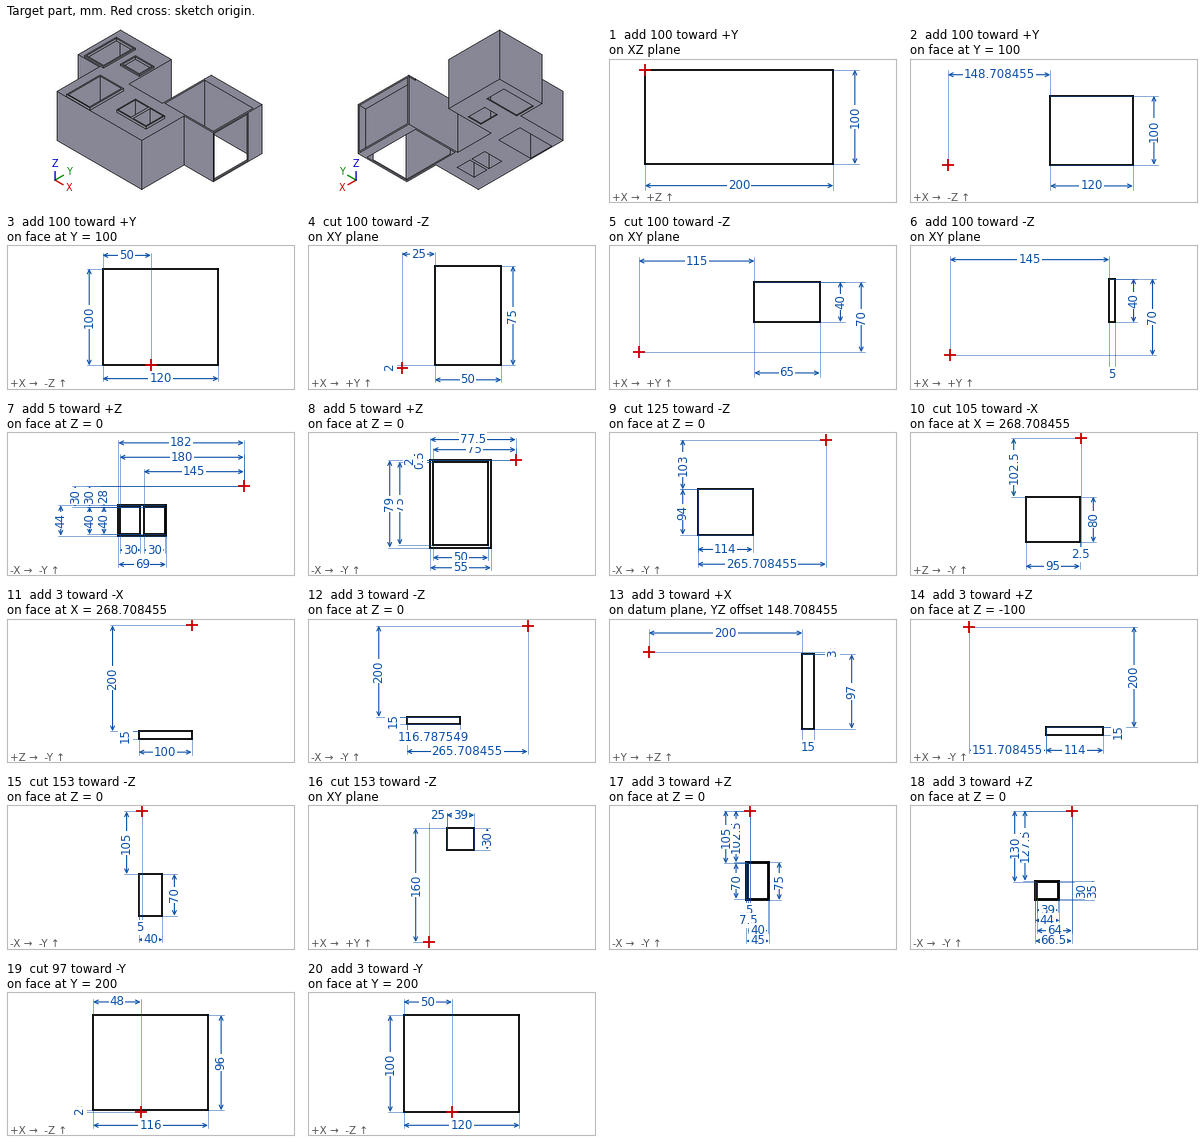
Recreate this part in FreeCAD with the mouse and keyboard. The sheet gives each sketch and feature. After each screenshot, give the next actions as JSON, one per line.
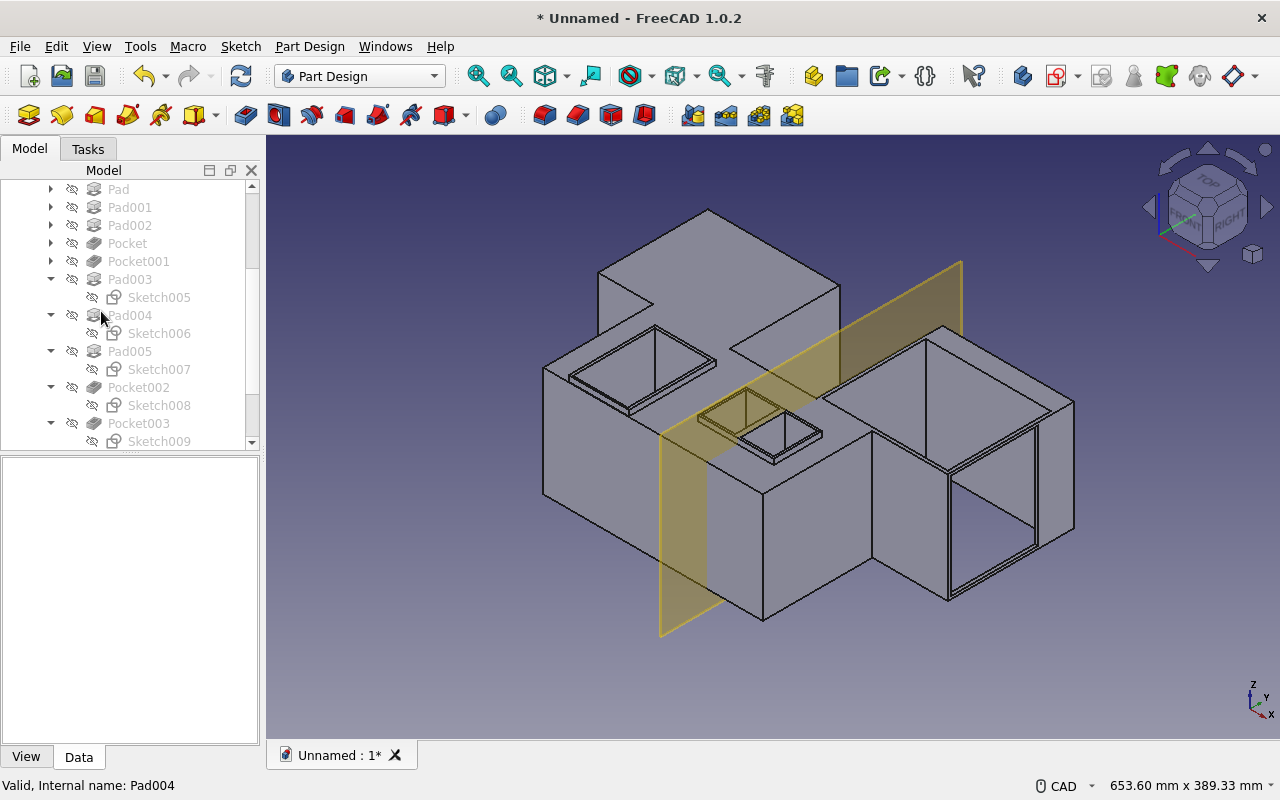
{"action": "scroll", "coordinate": [141, 311], "scroll_direction": "up", "scroll_amount": 15}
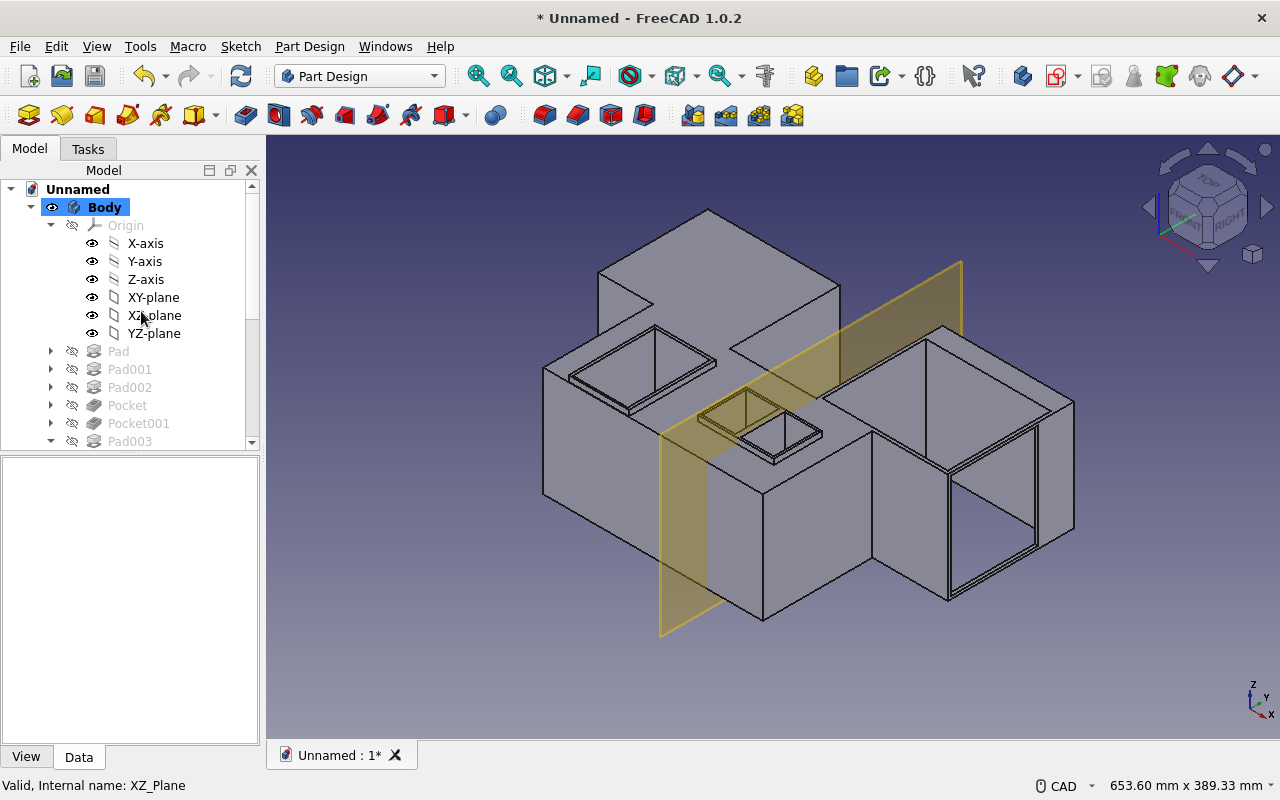
{"action": "scroll", "coordinate": [101, 311], "scroll_direction": "down", "scroll_amount": 6}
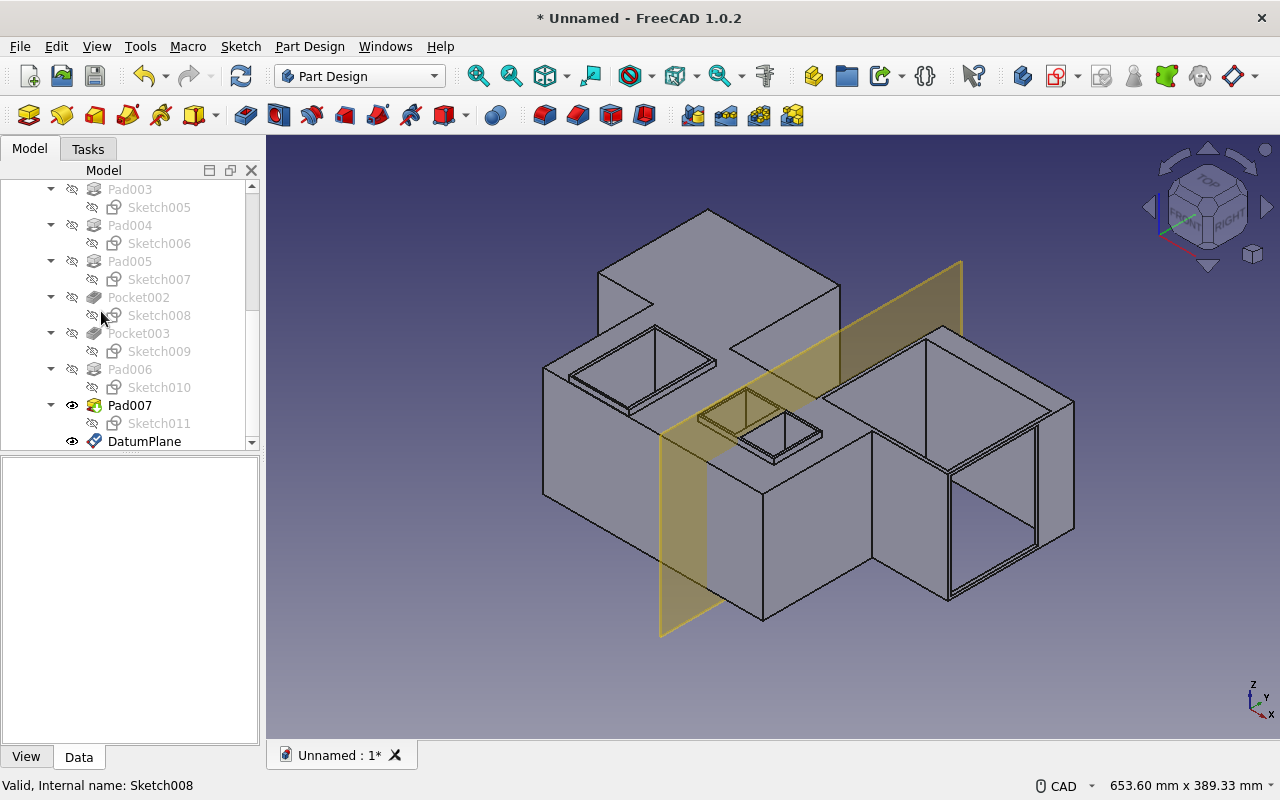
{"action": "left_click", "coordinate": [117, 441]}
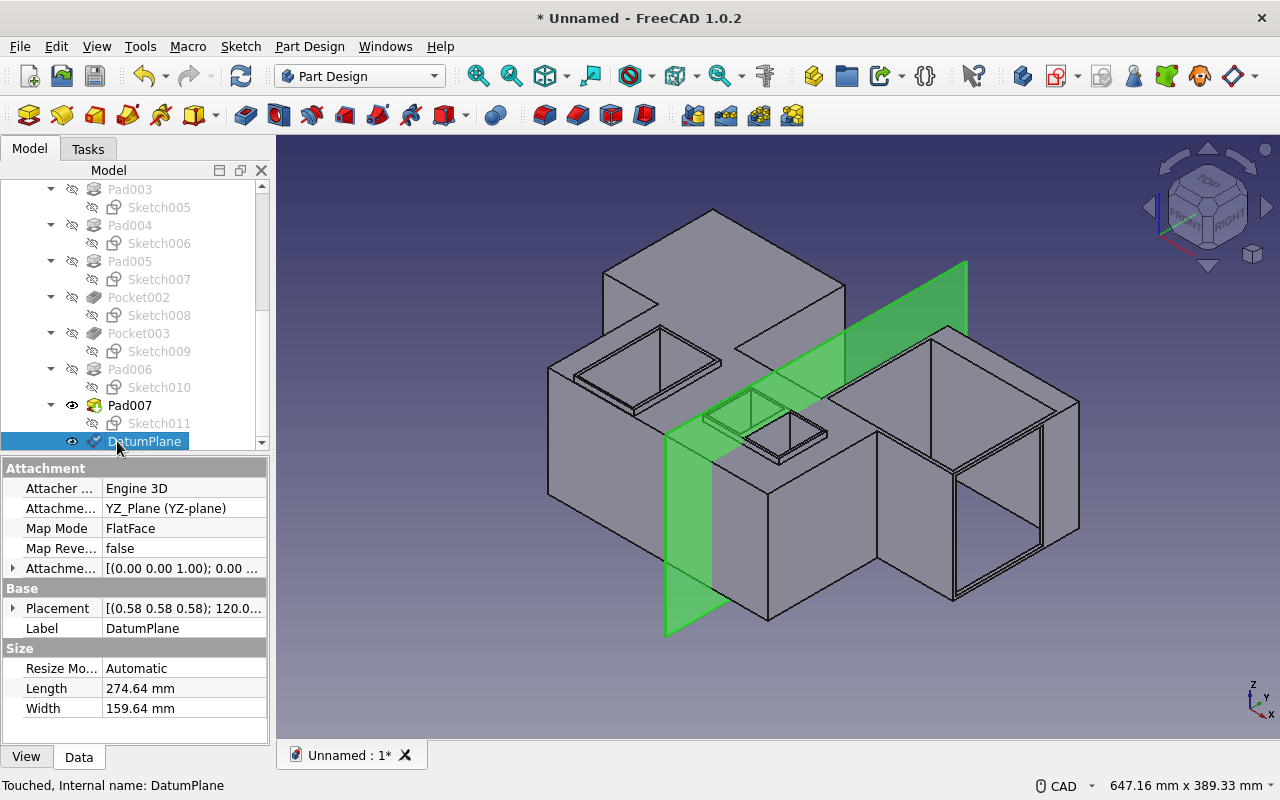
{"action": "left_click", "coordinate": [1056, 76]}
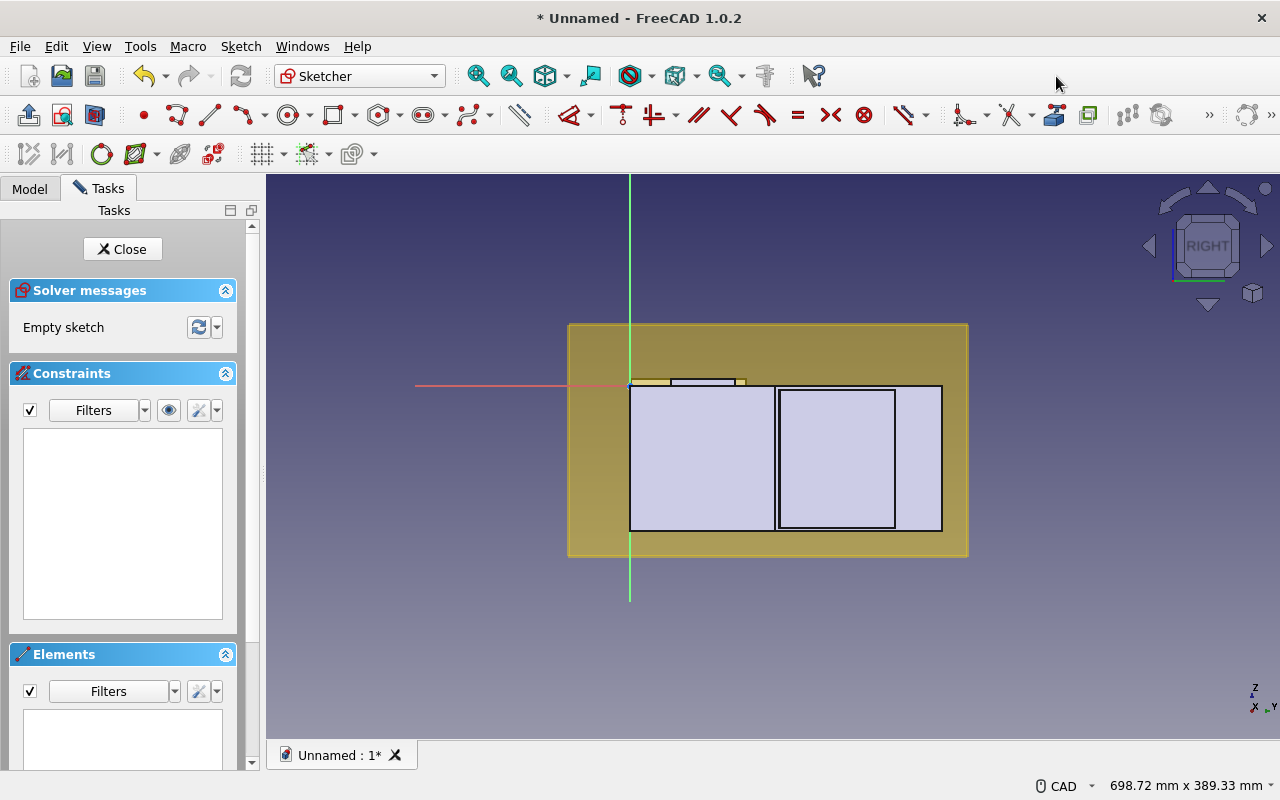
{"action": "left_click", "coordinate": [95, 116]}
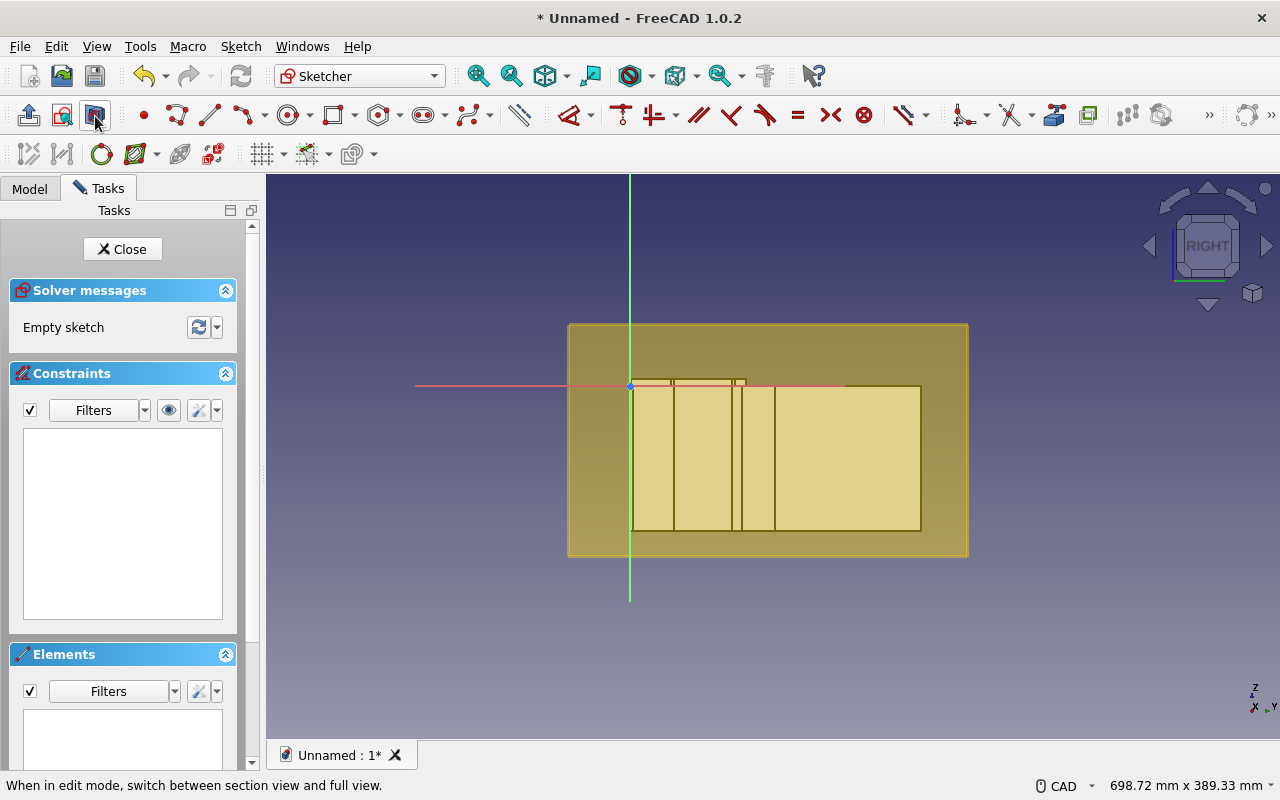
{"action": "scroll", "coordinate": [886, 462], "scroll_direction": "up", "scroll_amount": 3}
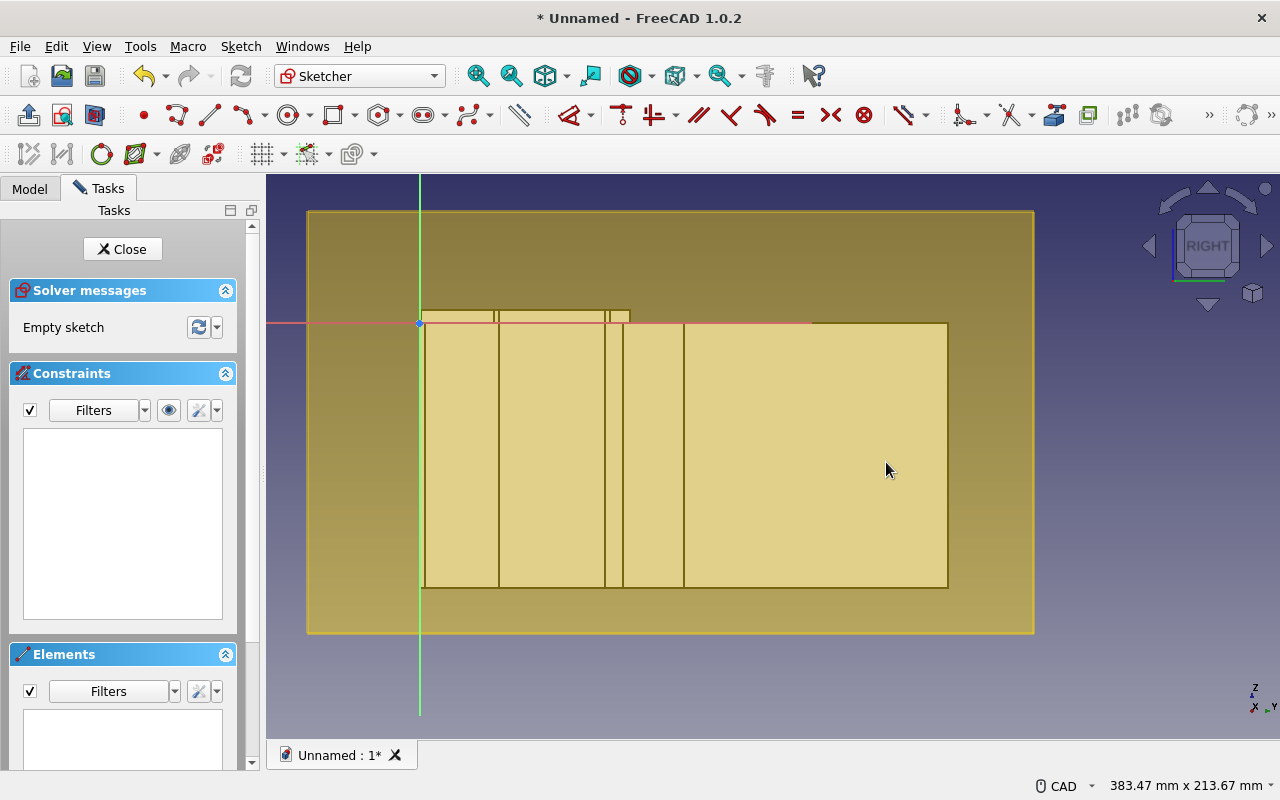
{"action": "left_click", "coordinate": [332, 116]}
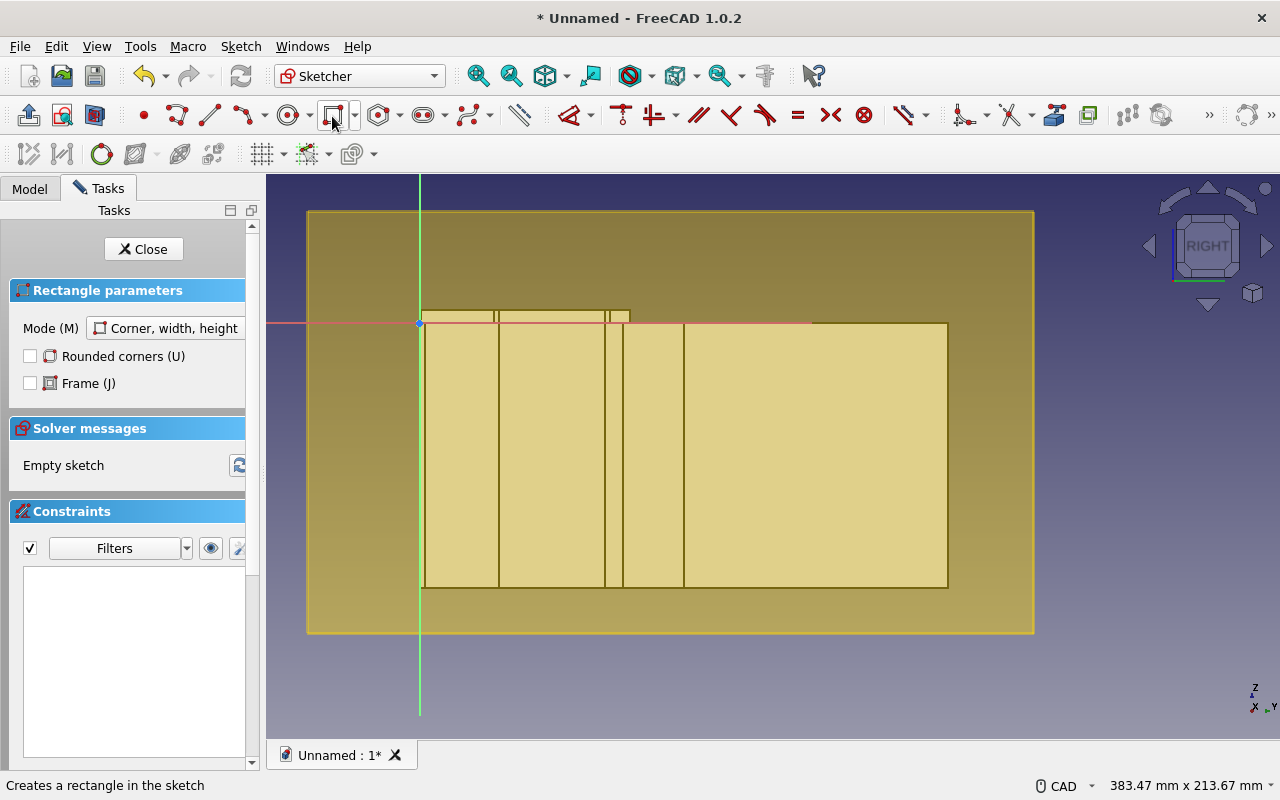
{"action": "scroll", "coordinate": [948, 331], "scroll_direction": "up", "scroll_amount": 4}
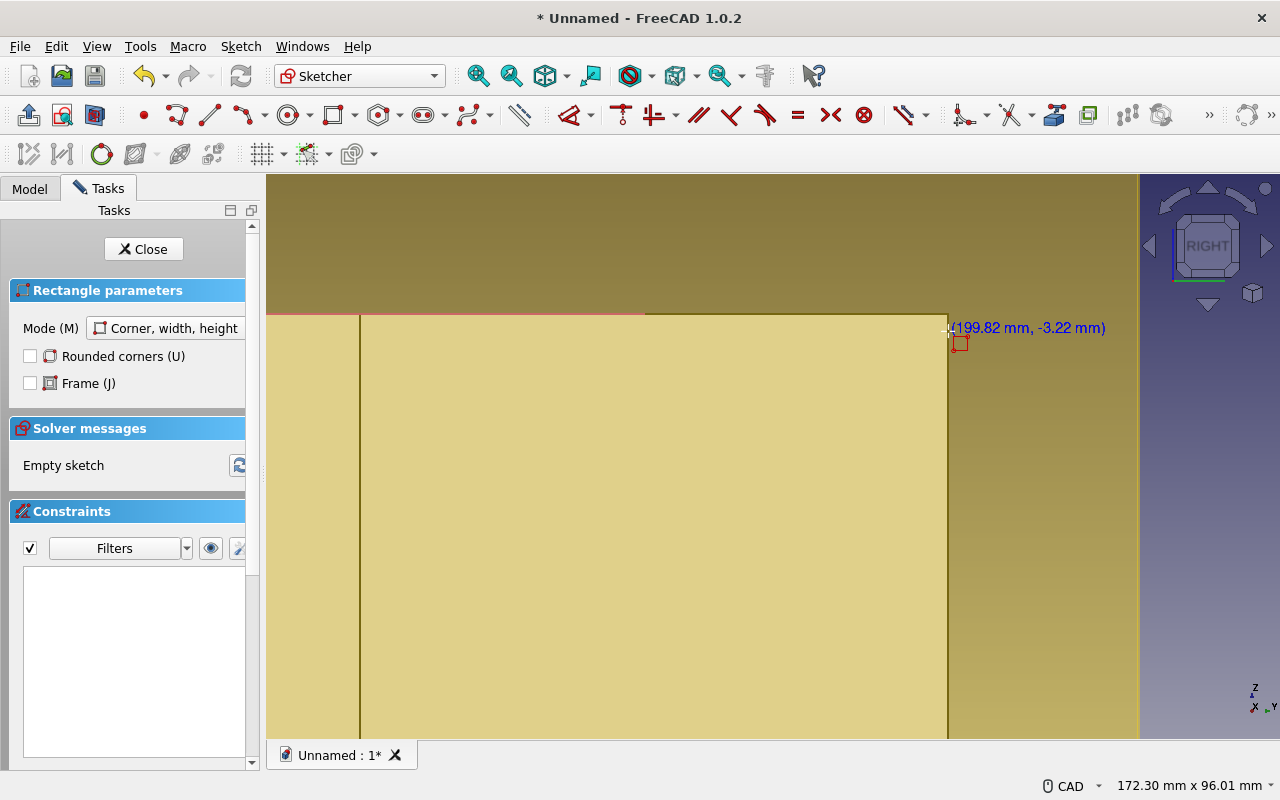
{"action": "left_click", "coordinate": [948, 332]}